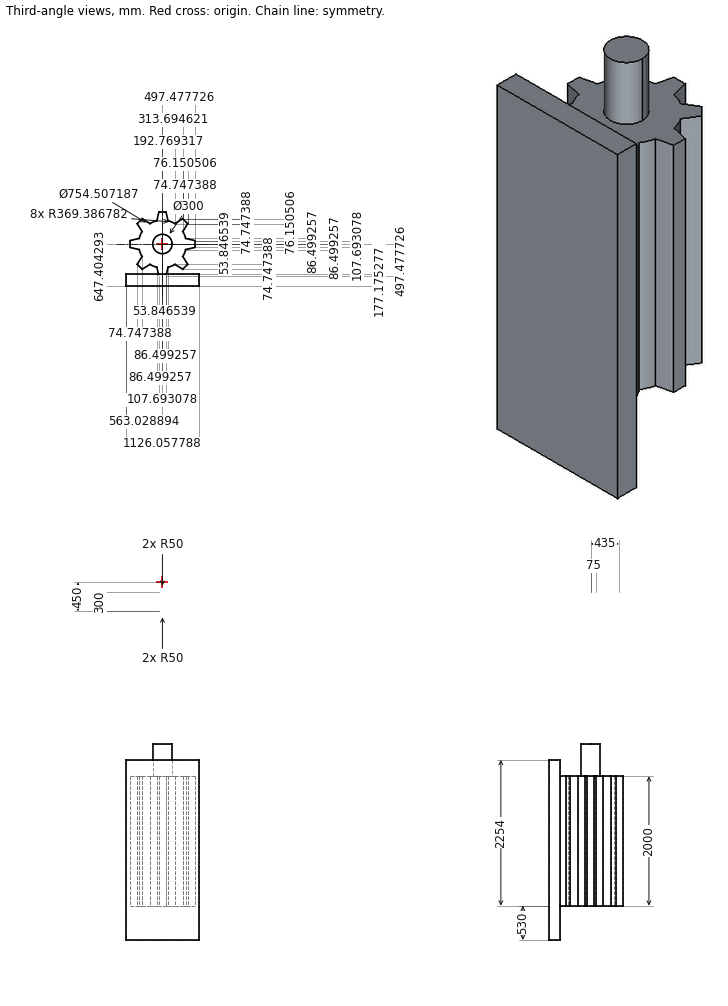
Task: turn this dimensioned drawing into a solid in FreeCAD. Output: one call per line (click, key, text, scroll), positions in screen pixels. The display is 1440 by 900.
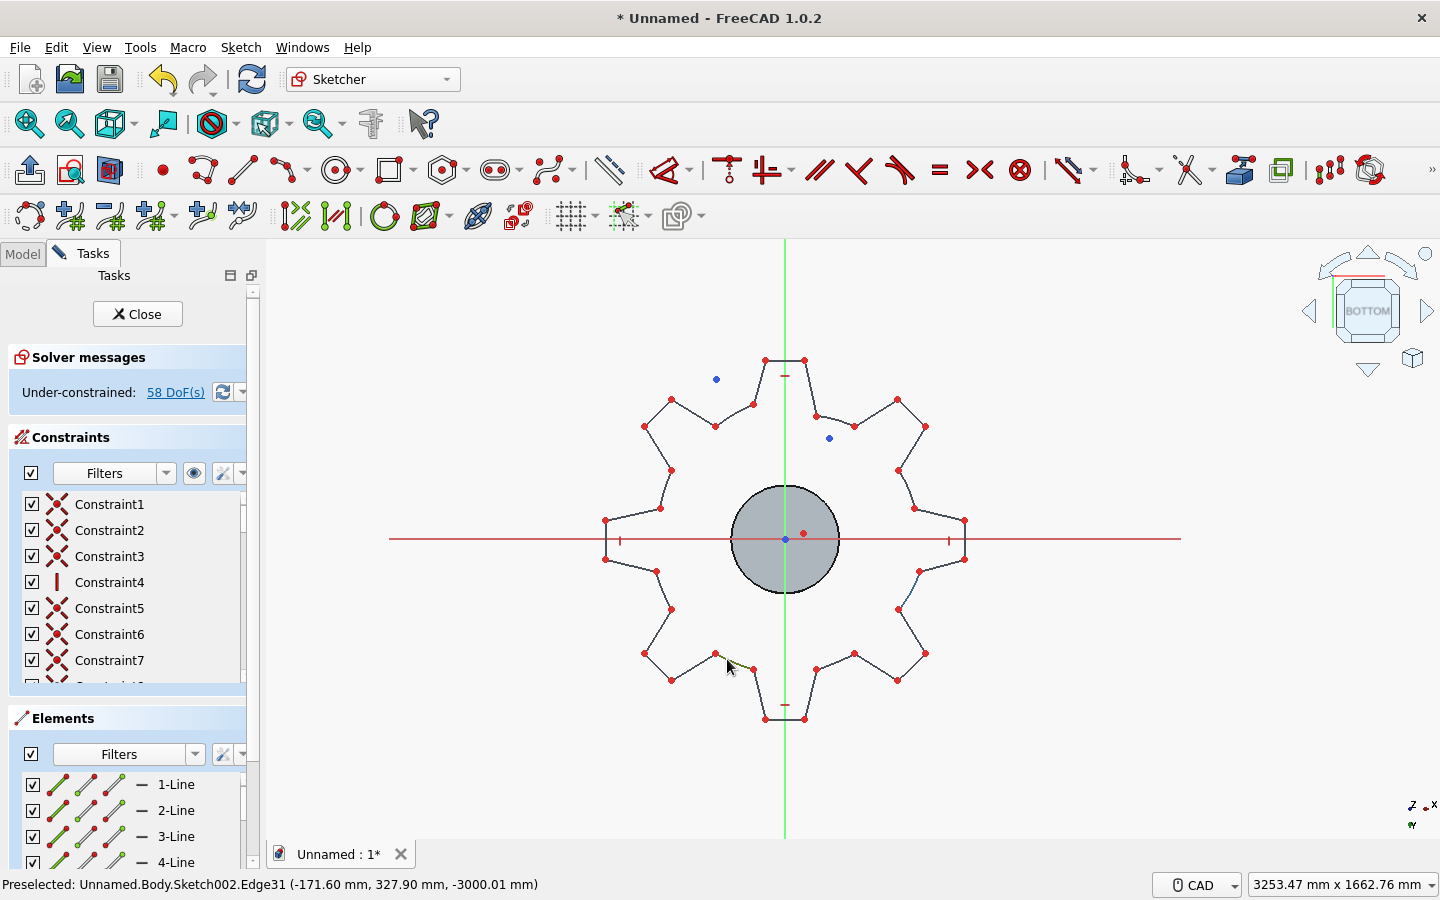
click(728, 170)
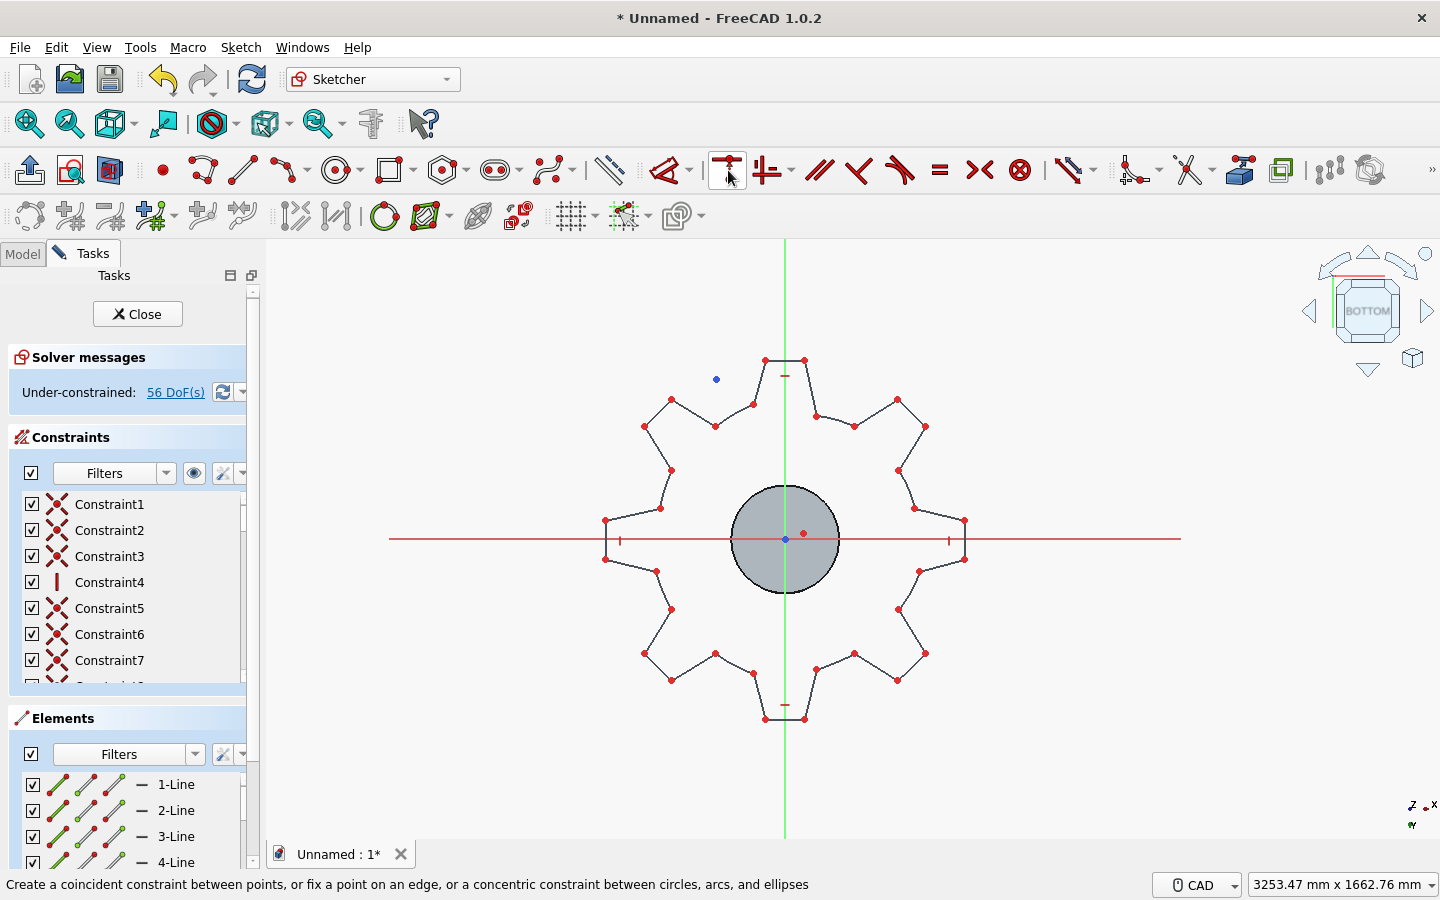
click(907, 599)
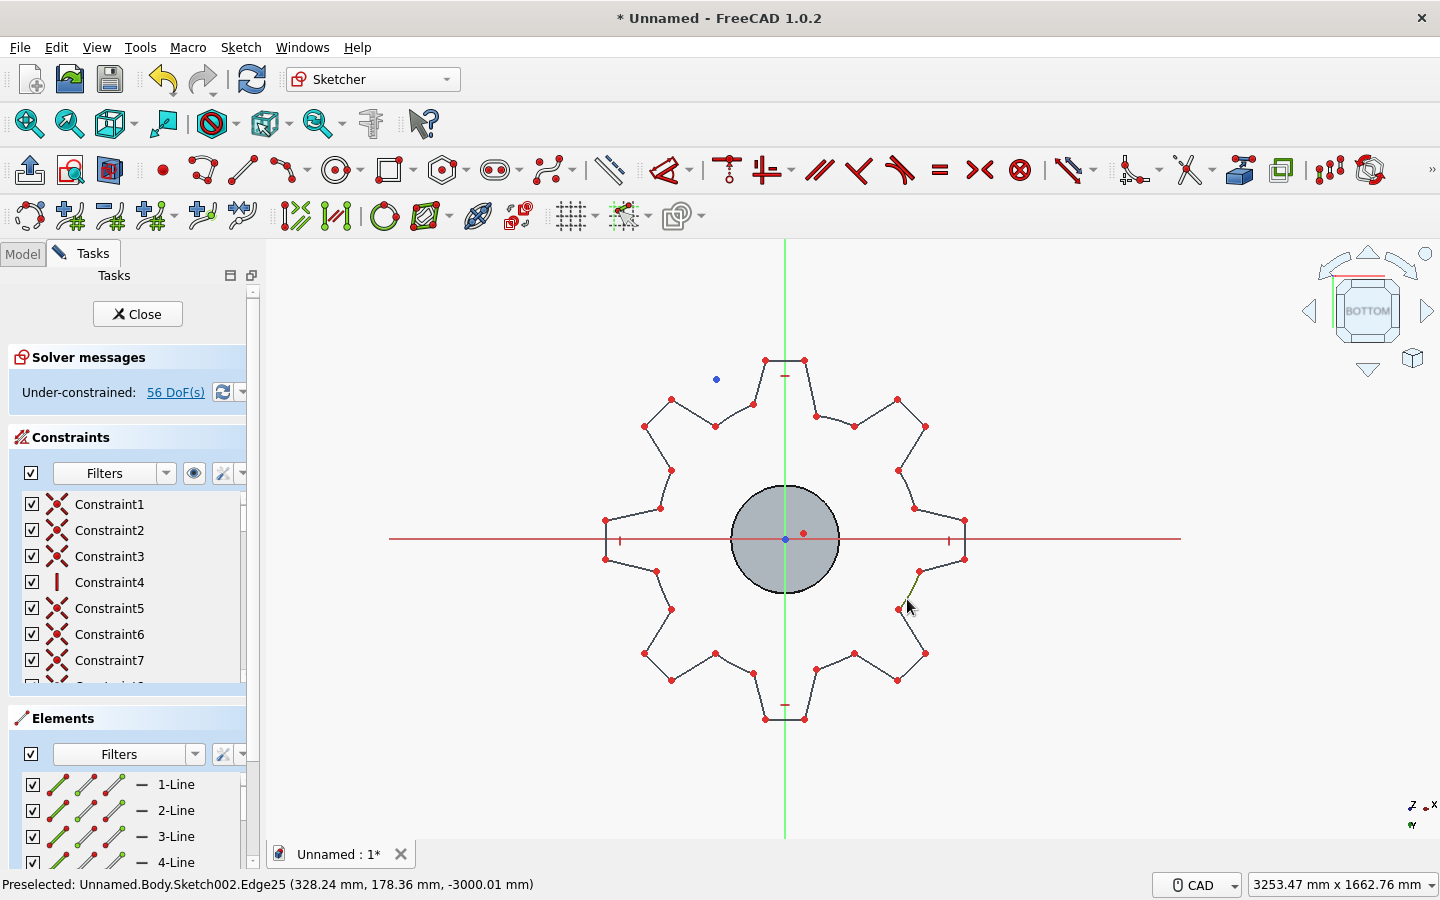
click(829, 666)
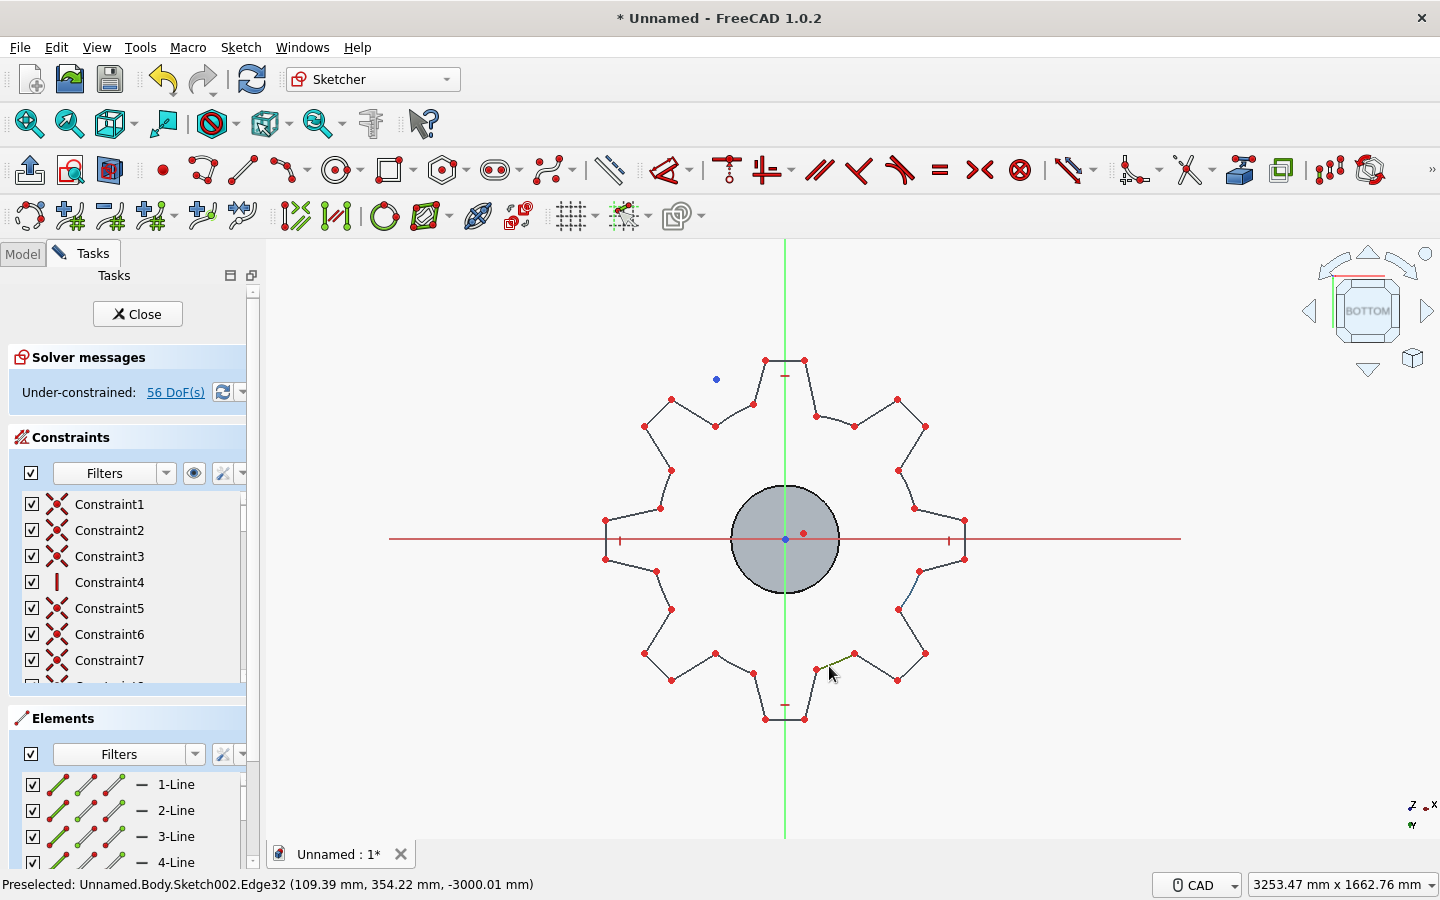
click(728, 170)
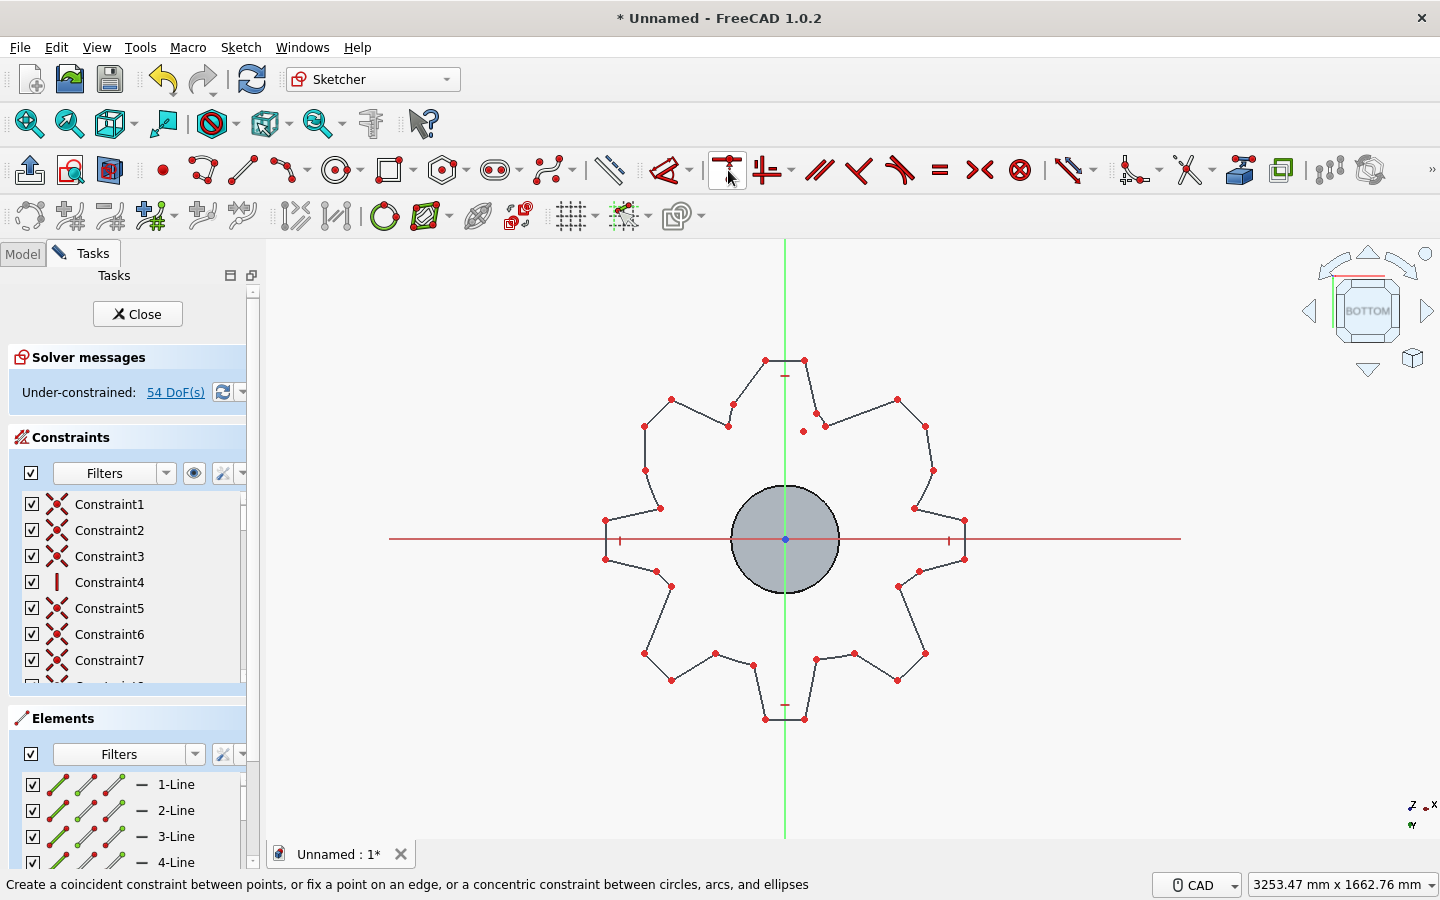
scroll(795, 485, up, 3)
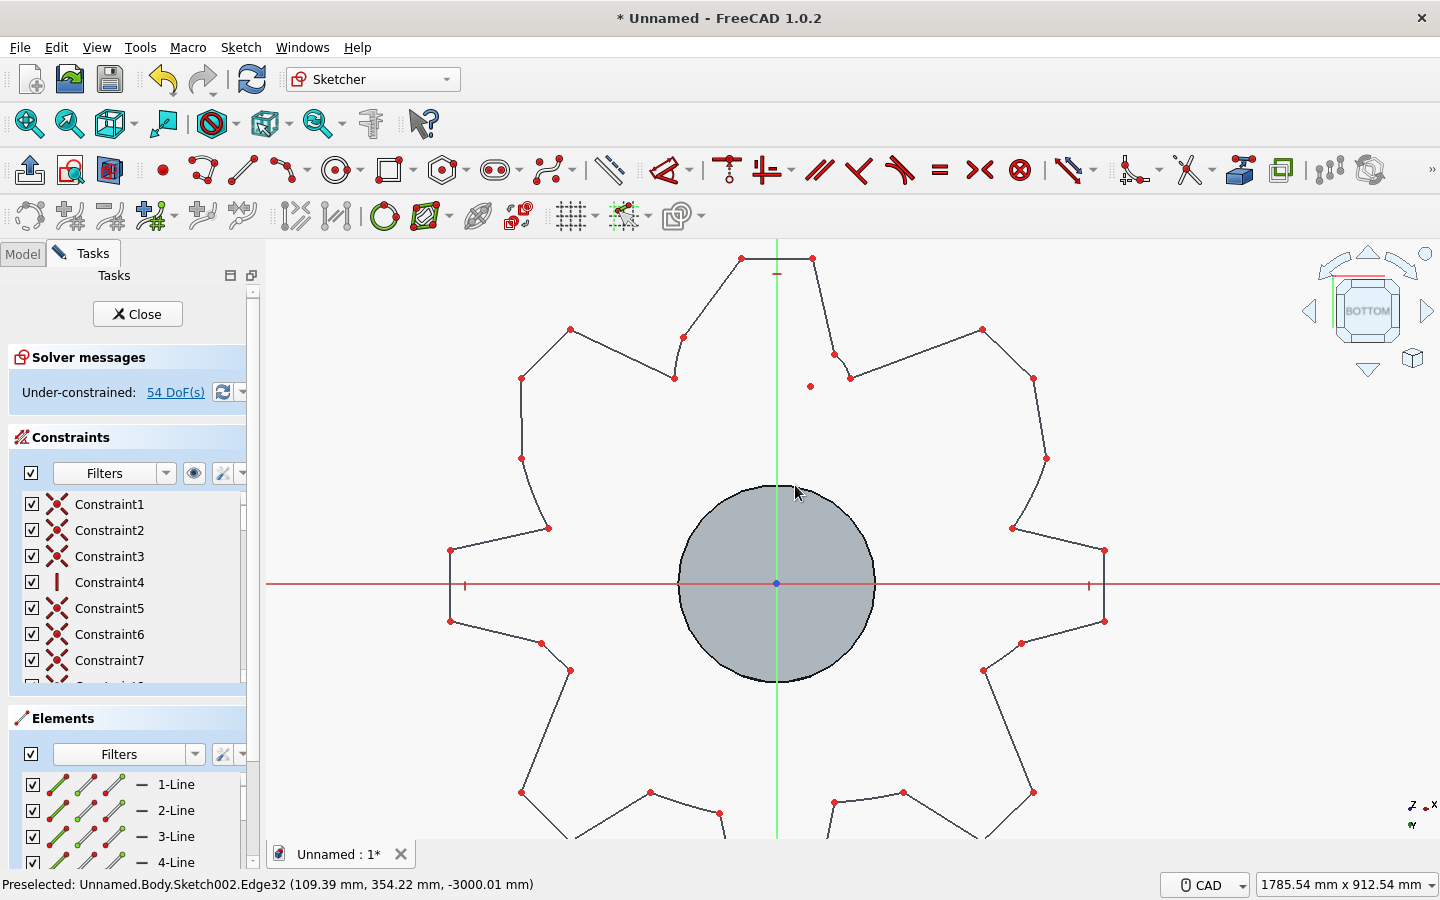
drag(767, 377, 821, 594)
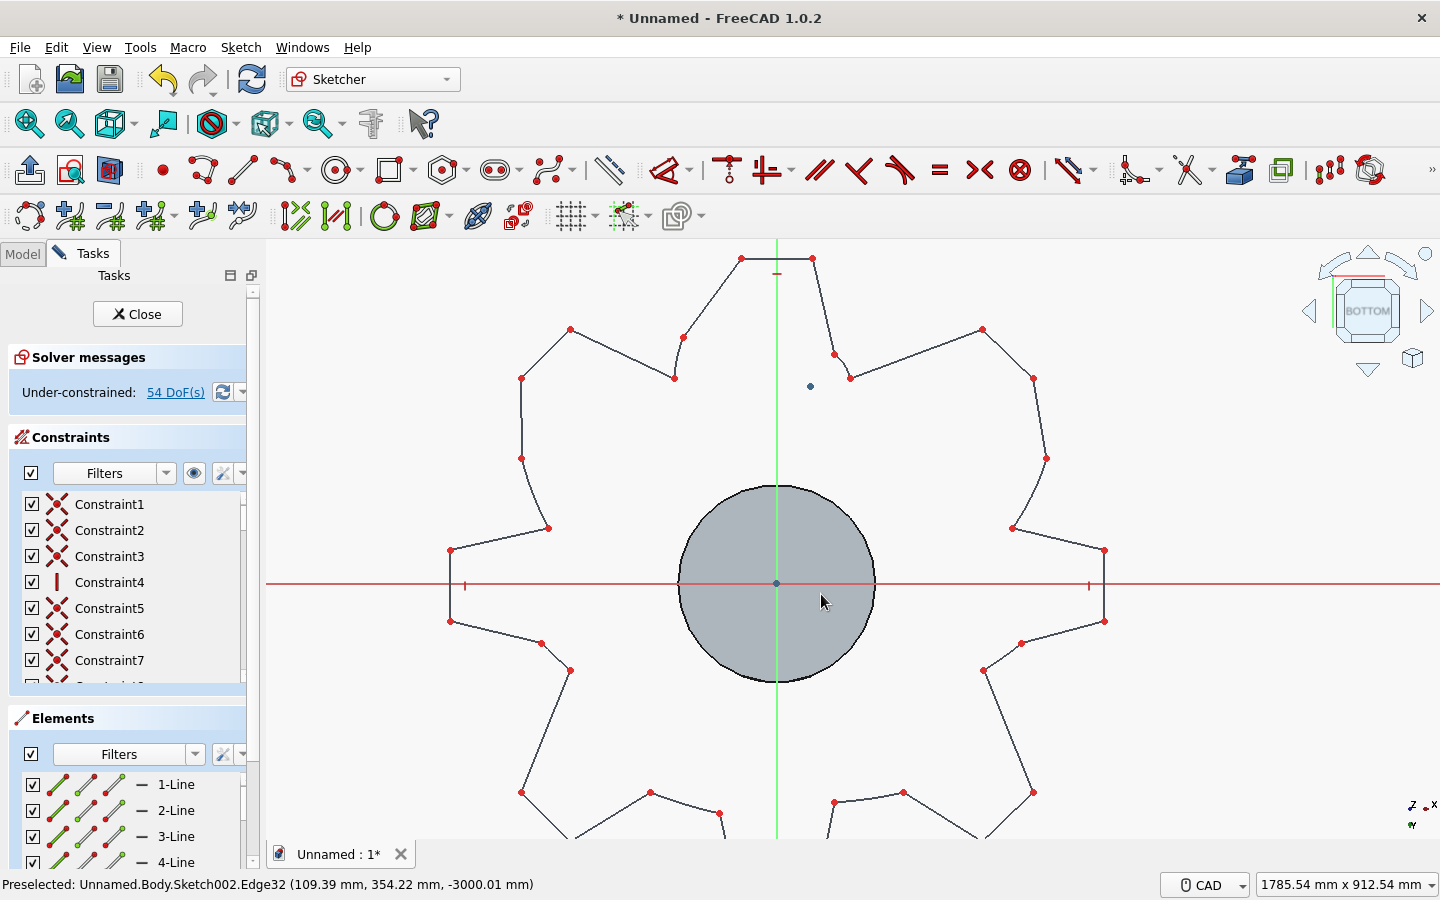
click(728, 170)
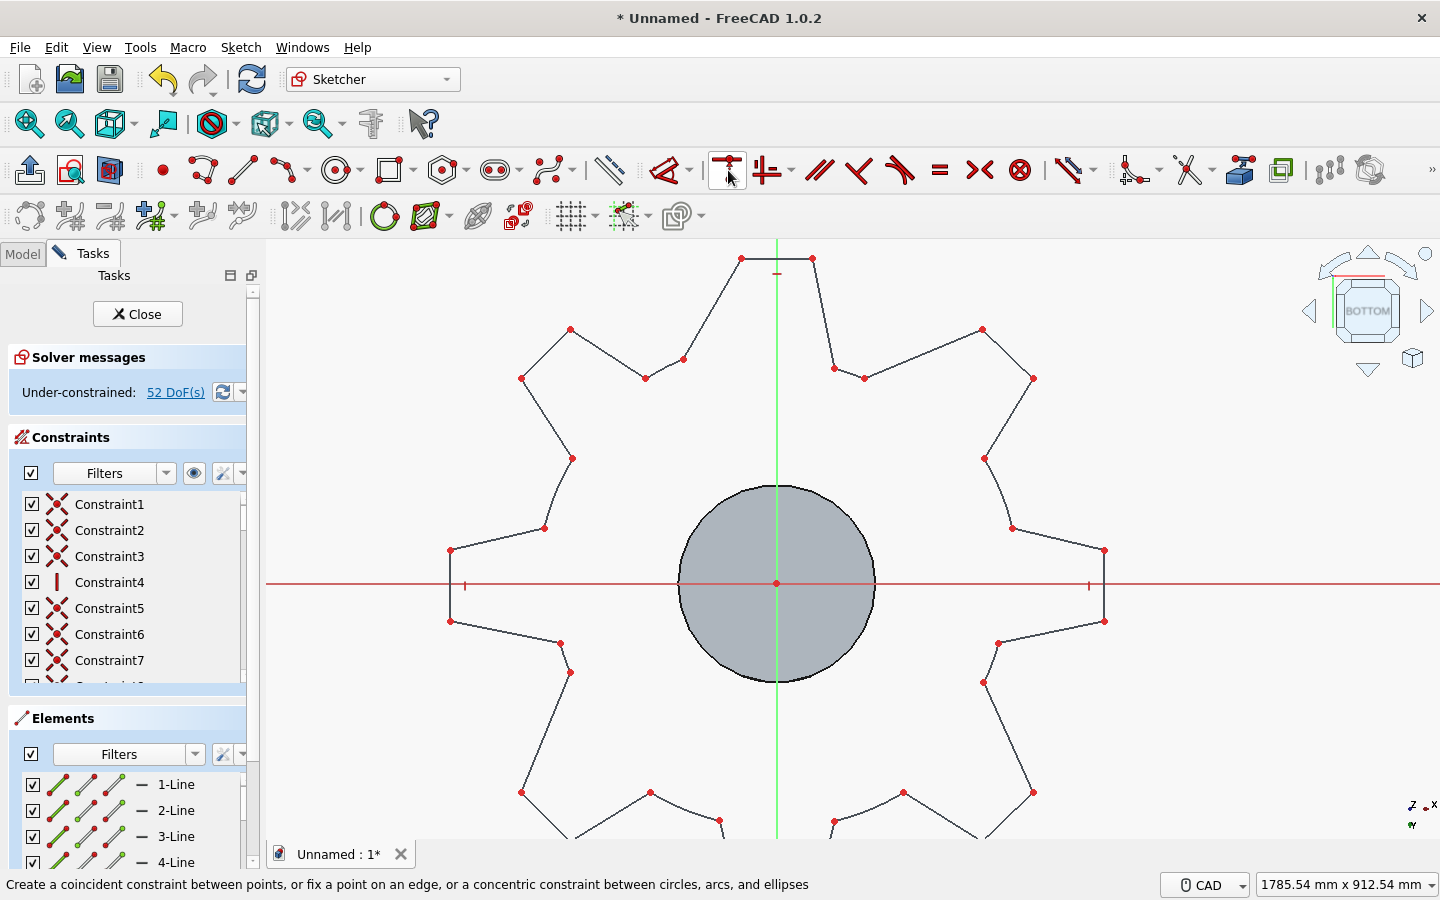
click(989, 671)